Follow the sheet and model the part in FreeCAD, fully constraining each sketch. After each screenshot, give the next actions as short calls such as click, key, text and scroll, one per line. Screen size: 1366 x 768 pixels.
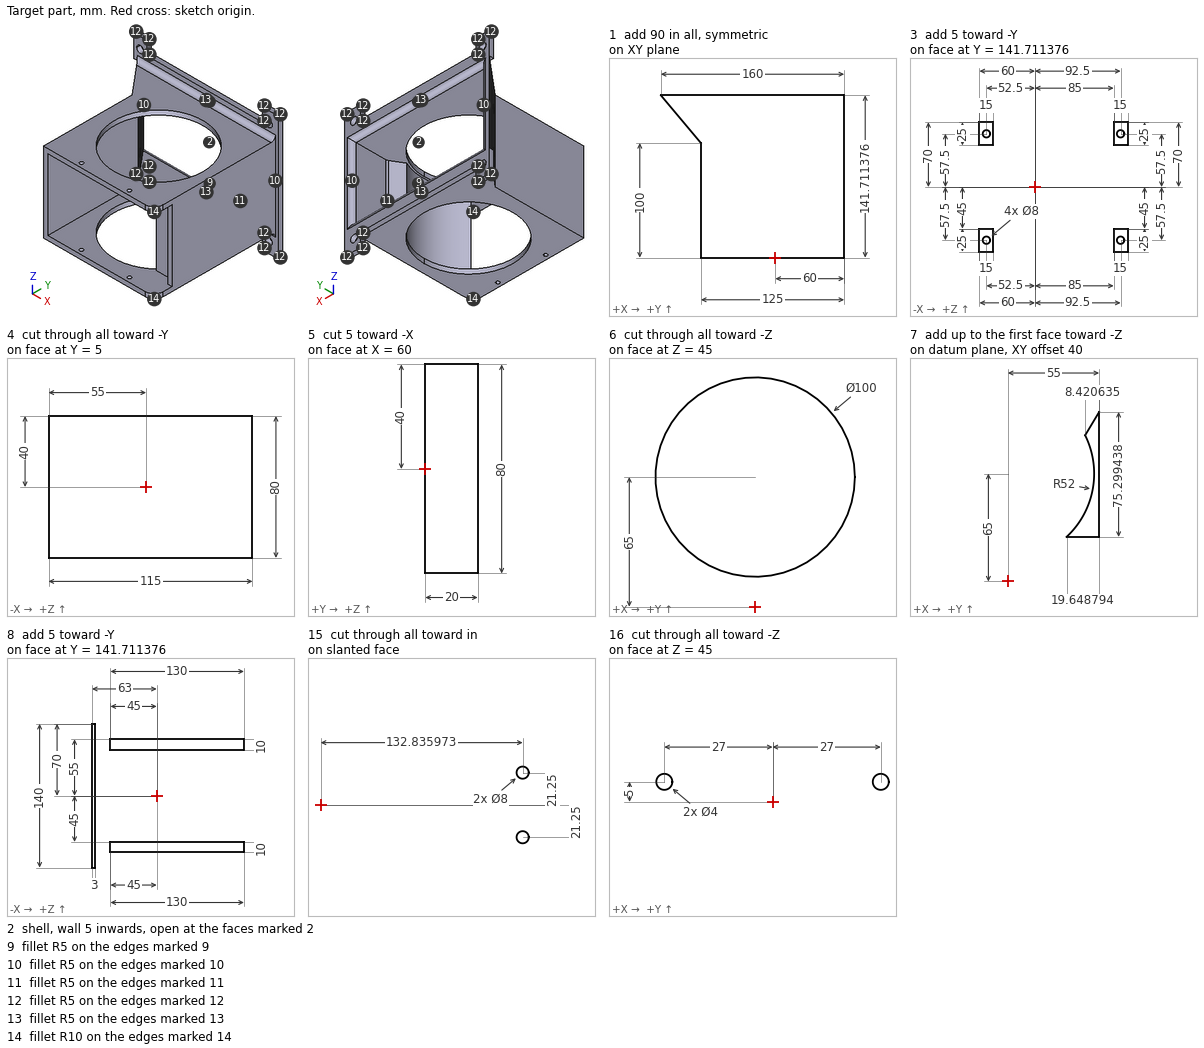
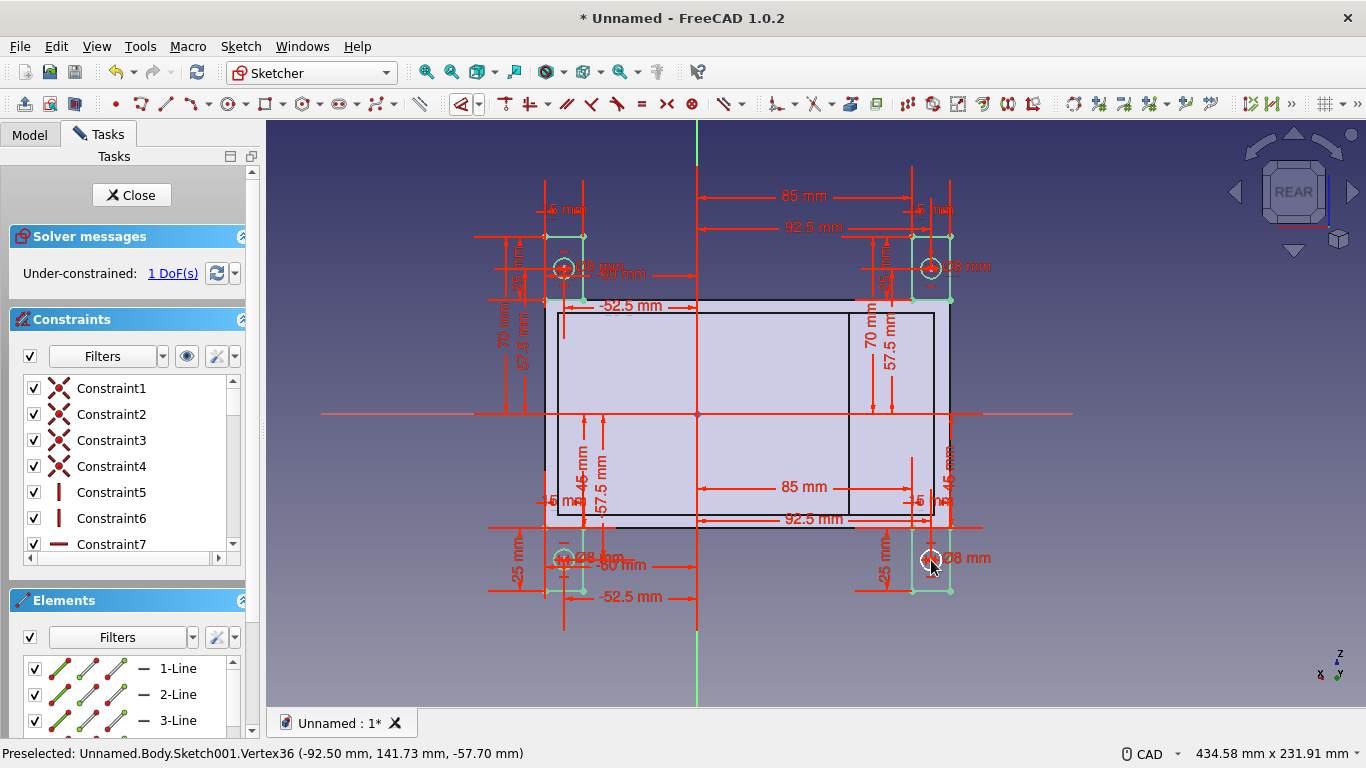
click(478, 104)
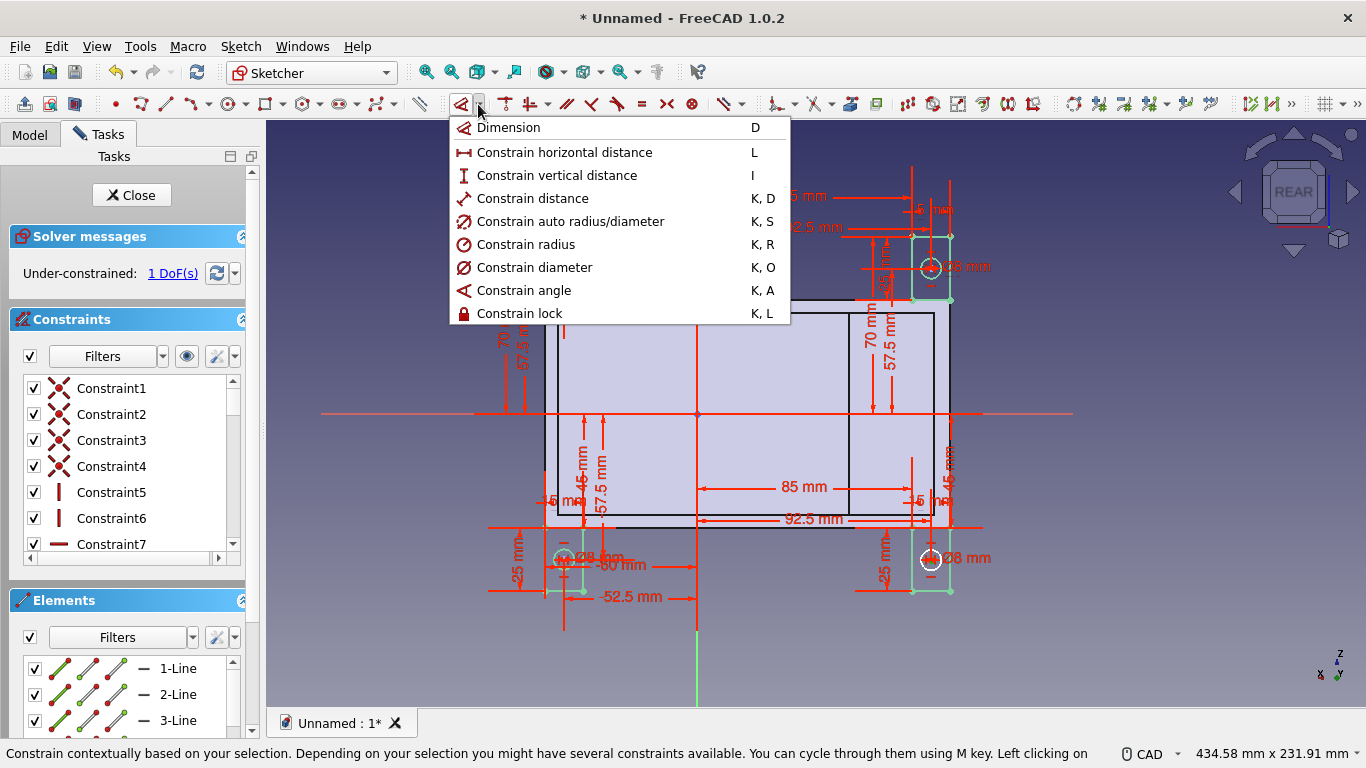
click(620, 176)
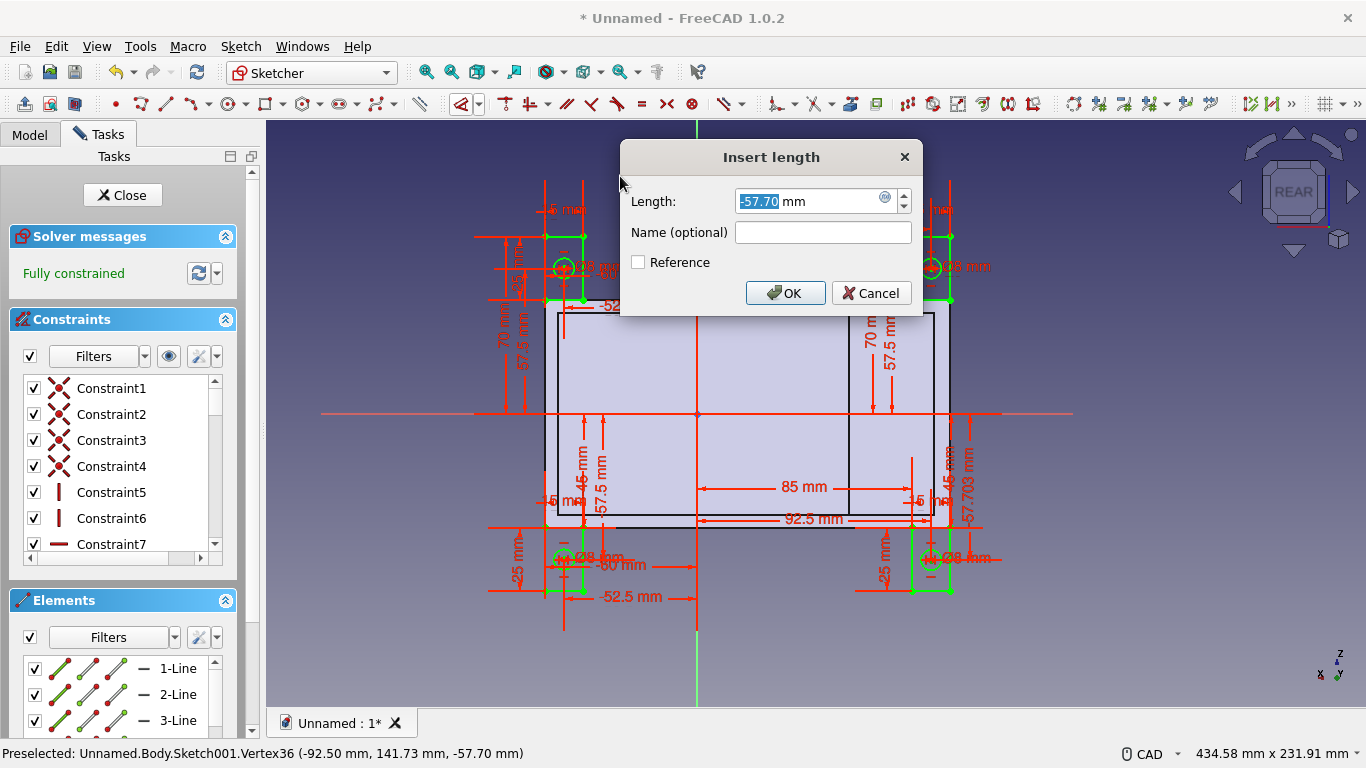
text(-57.5)
key(Return)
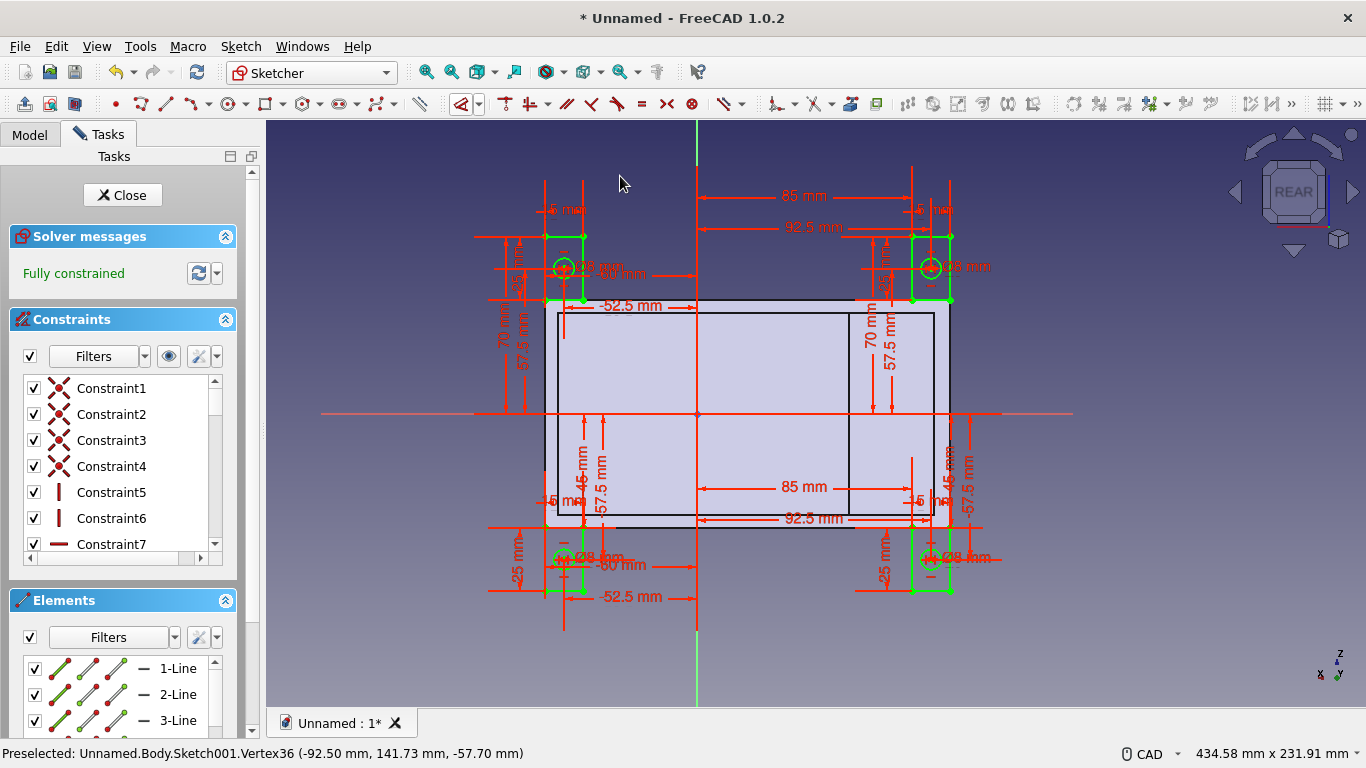
click(123, 195)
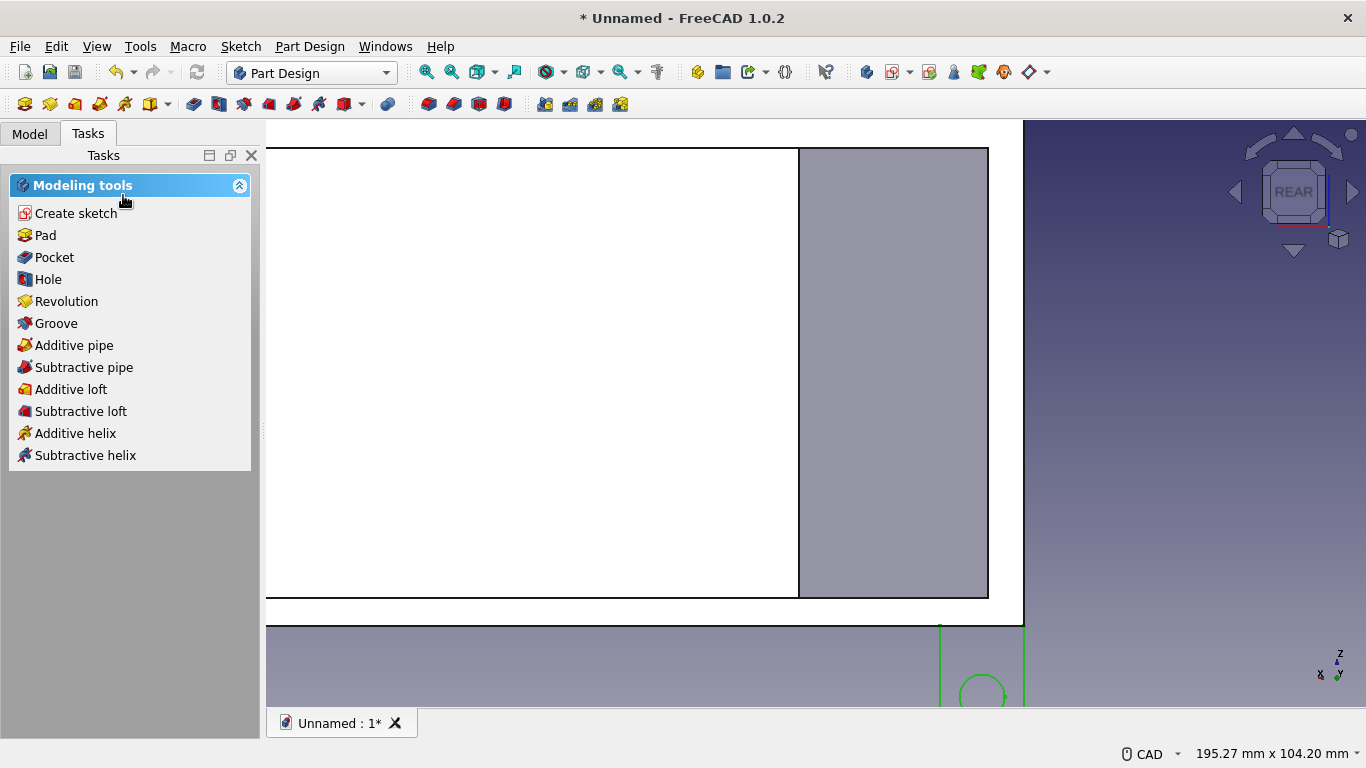
click(25, 104)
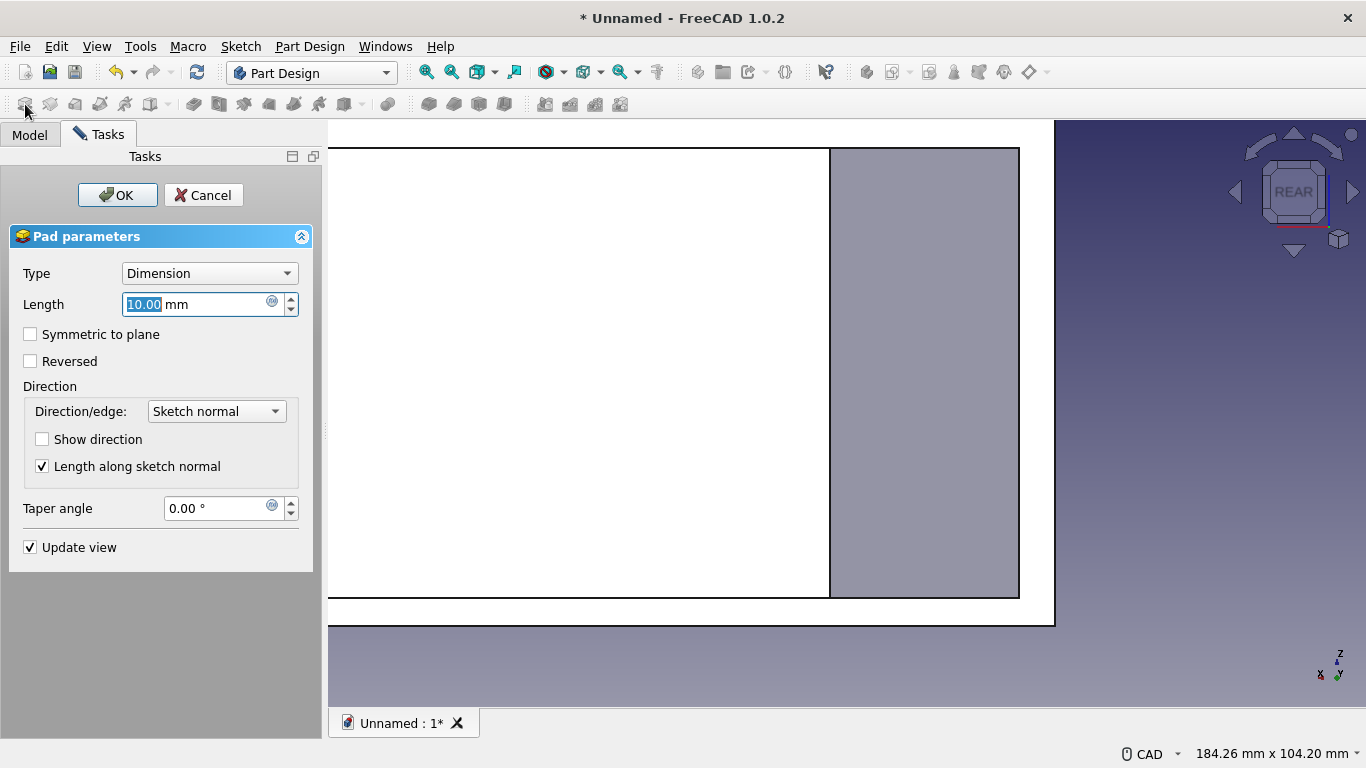
text(5)
key(Tab)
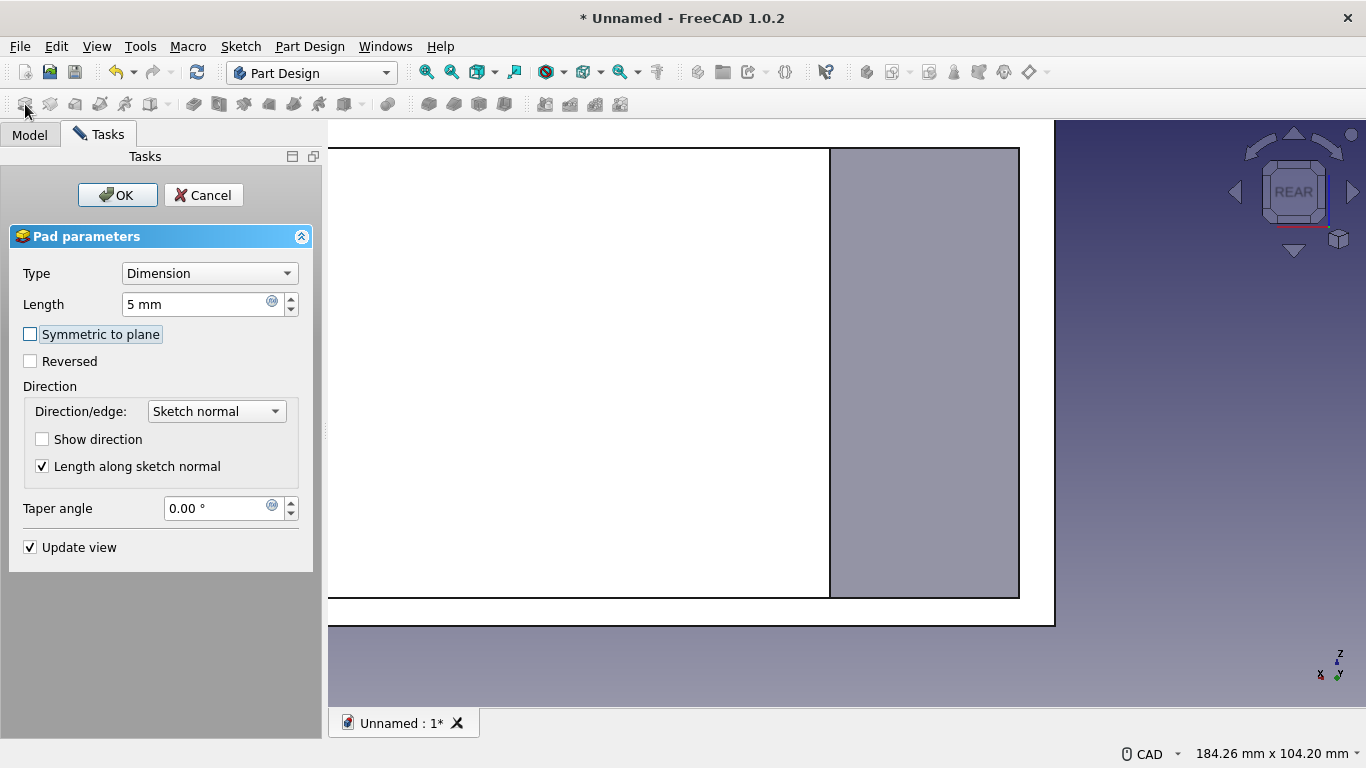
click(31, 361)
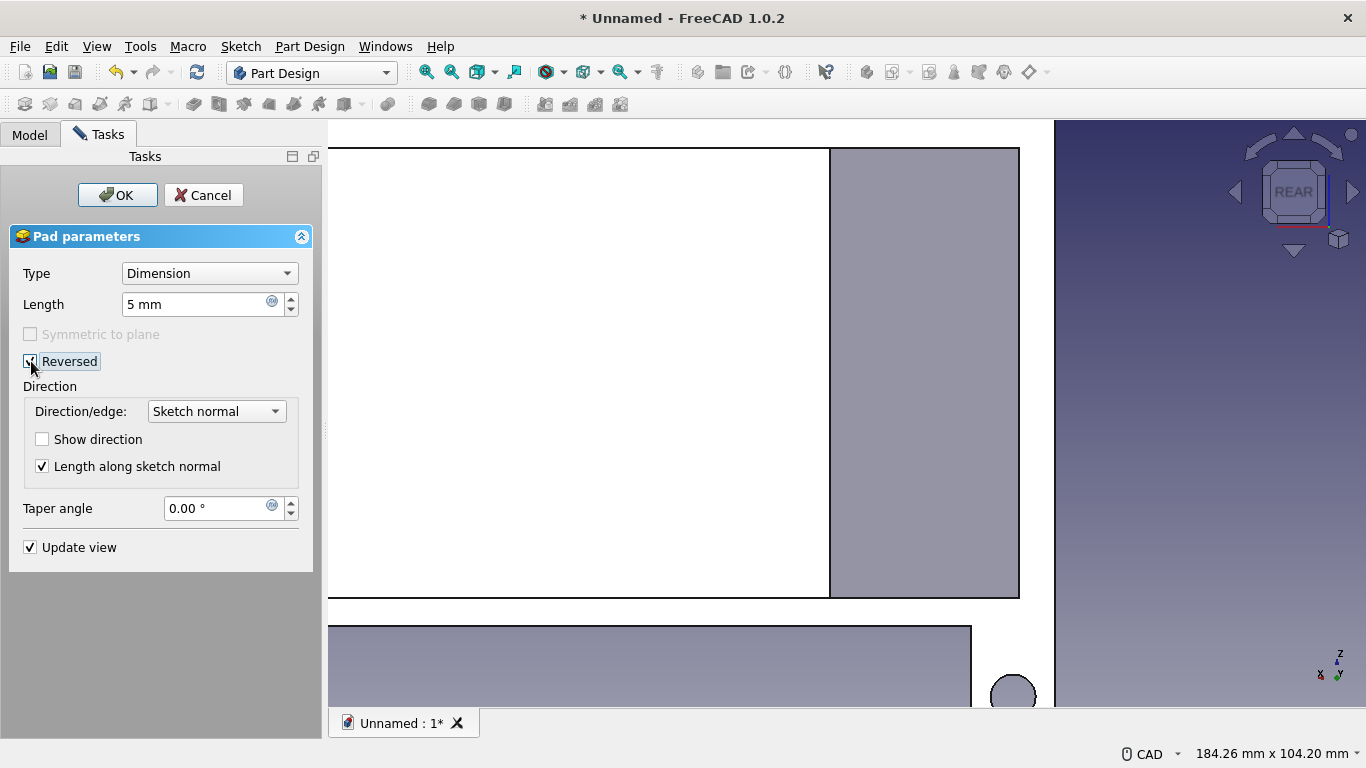
click(118, 195)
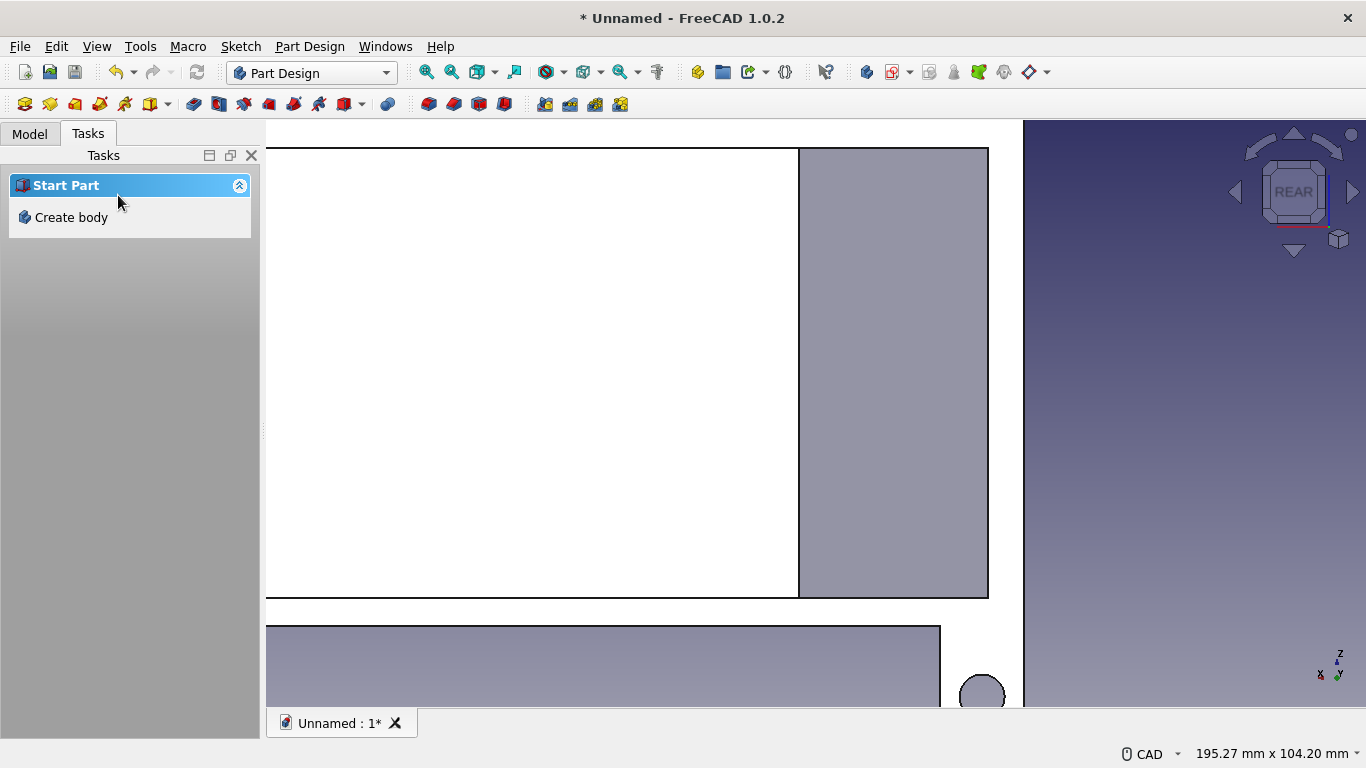
key(v)
key(f)